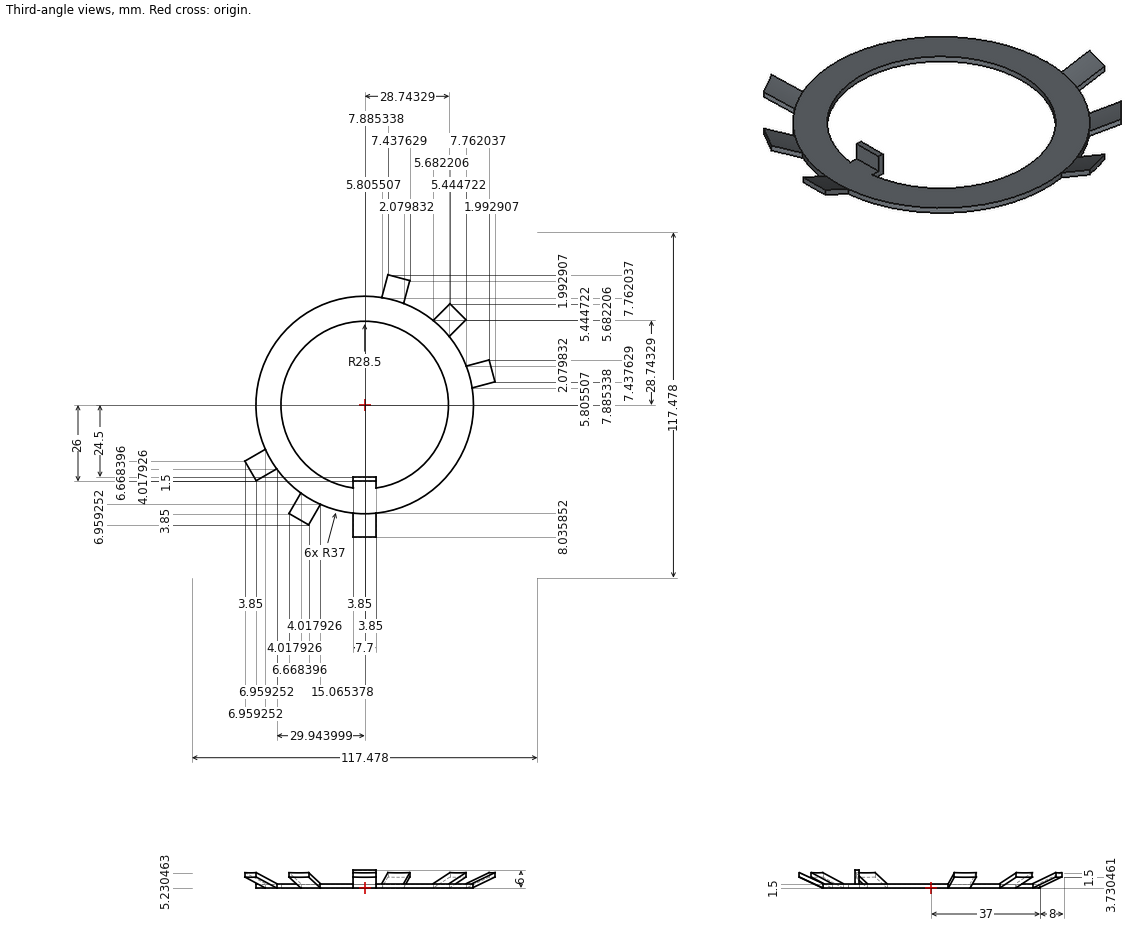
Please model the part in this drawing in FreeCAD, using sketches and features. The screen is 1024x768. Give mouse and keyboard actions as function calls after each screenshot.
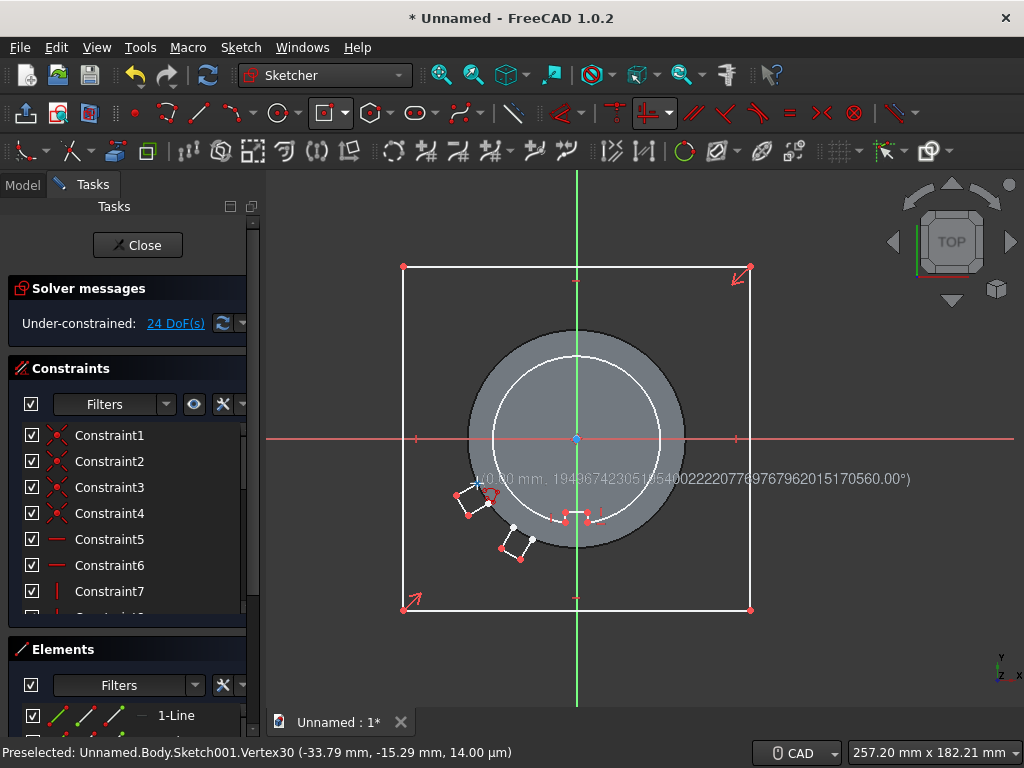
click(594, 331)
click(600, 308)
click(622, 314)
click(616, 337)
right_click(616, 337)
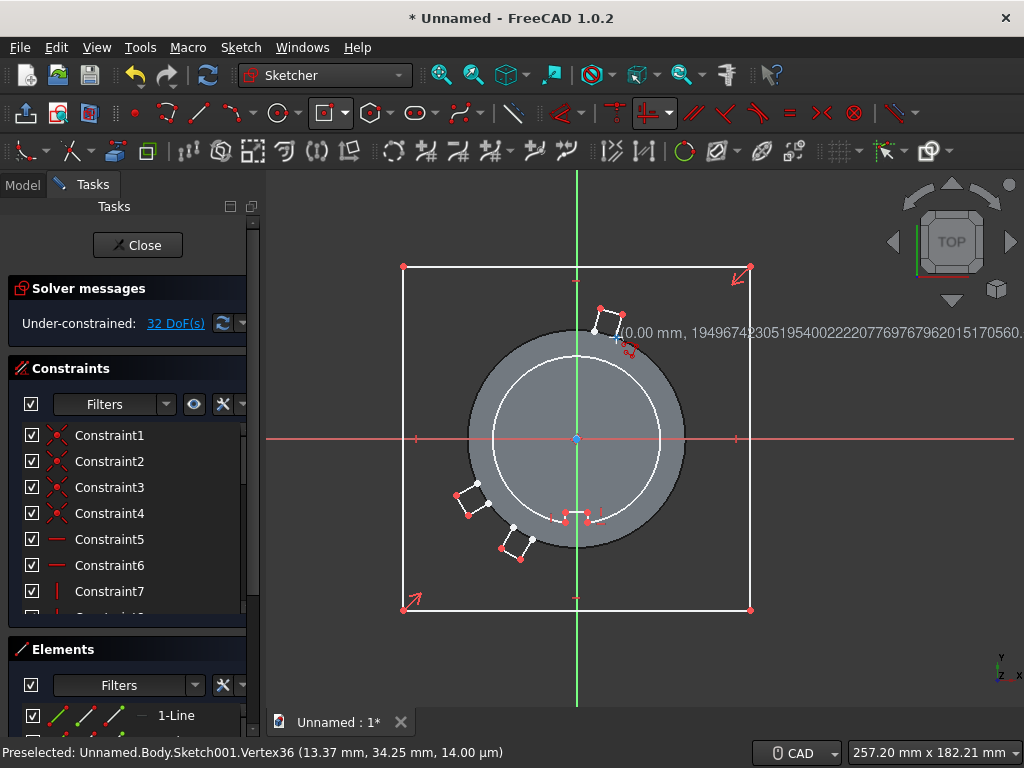
click(645, 354)
click(662, 337)
click(678, 354)
click(661, 370)
right_click(661, 370)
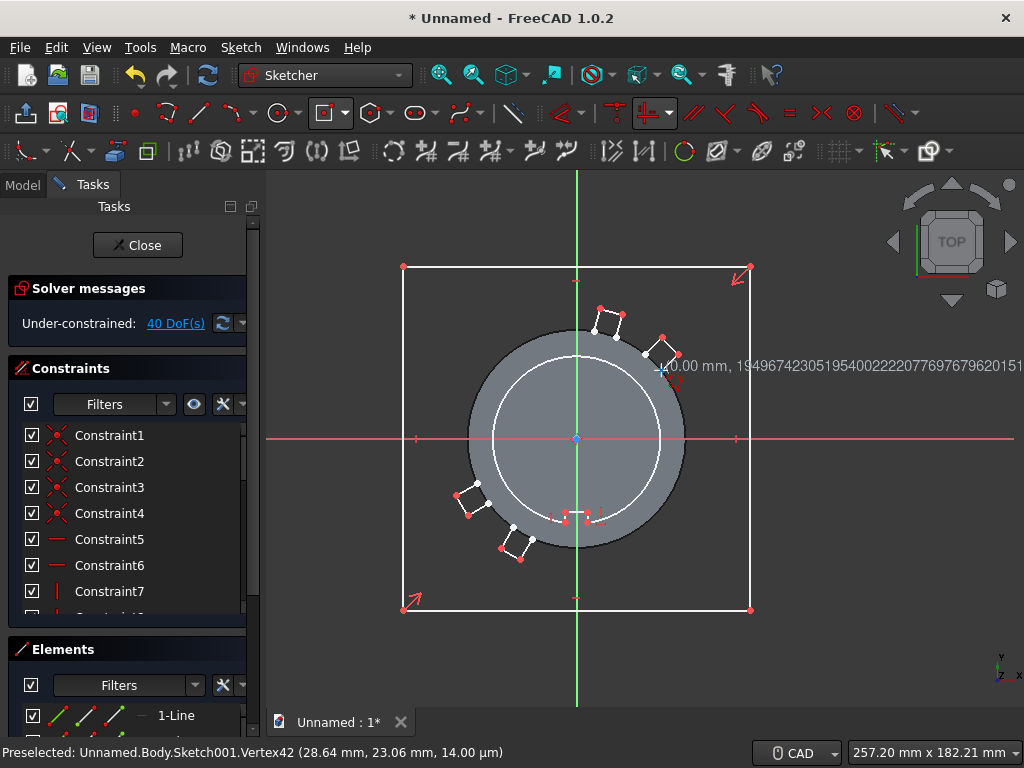
click(678, 400)
click(701, 394)
click(707, 416)
click(684, 422)
right_click(684, 422)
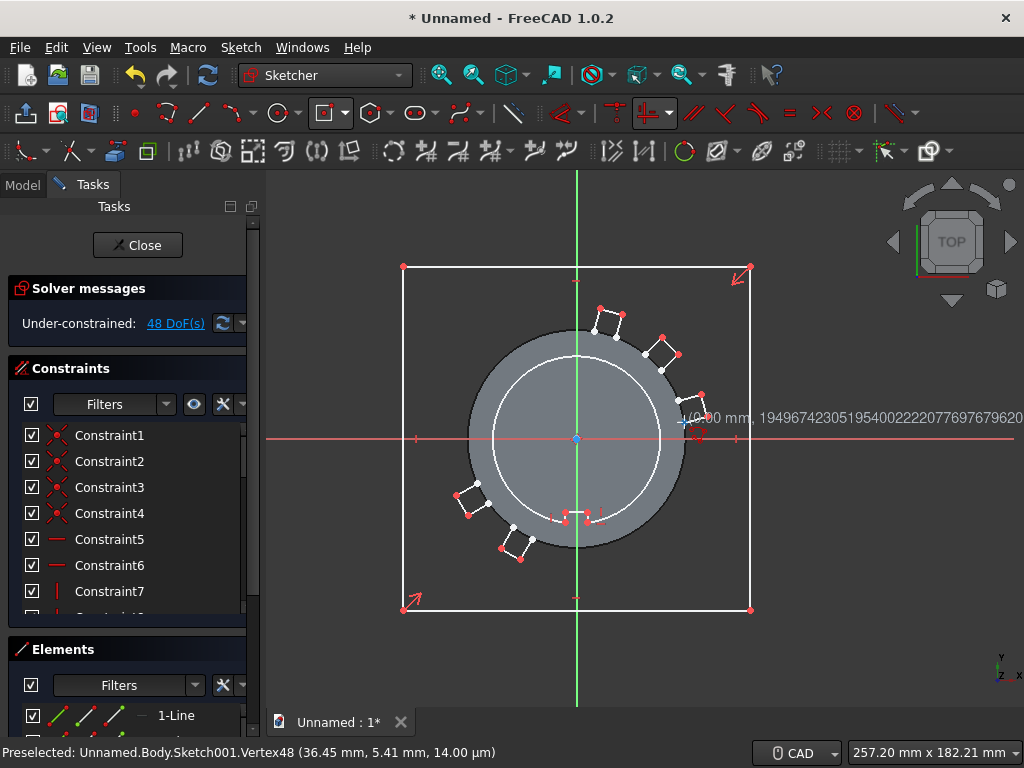
scroll(588, 547, up, 2)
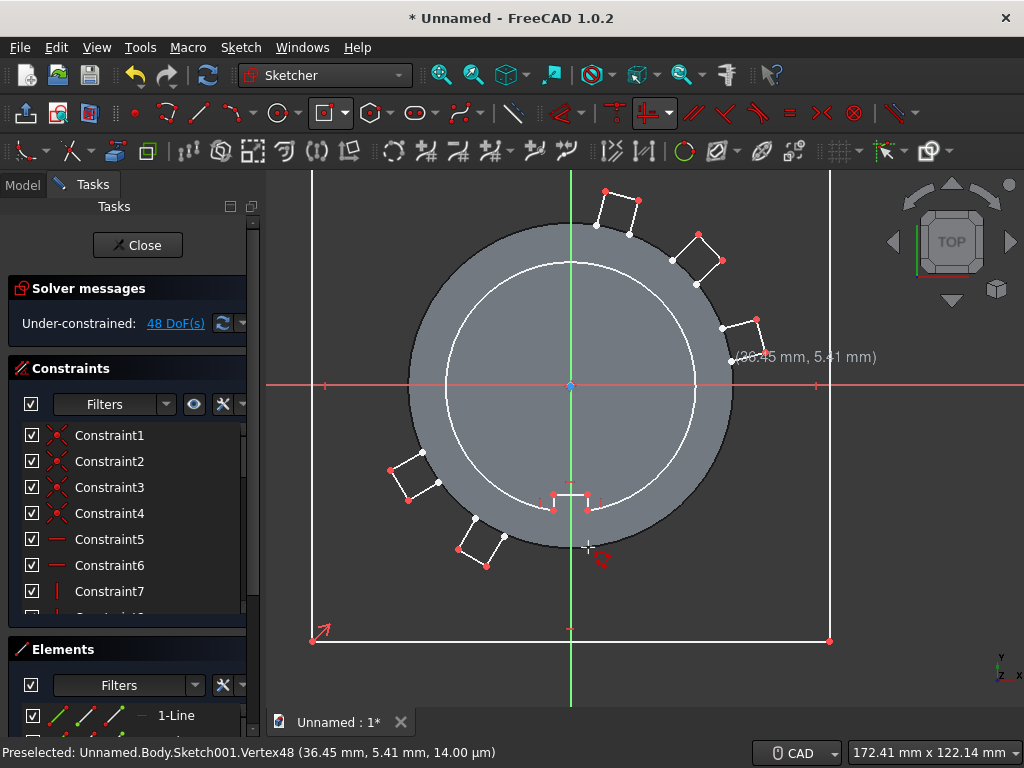
click(588, 547)
click(588, 583)
click(554, 583)
click(554, 547)
right_click(554, 547)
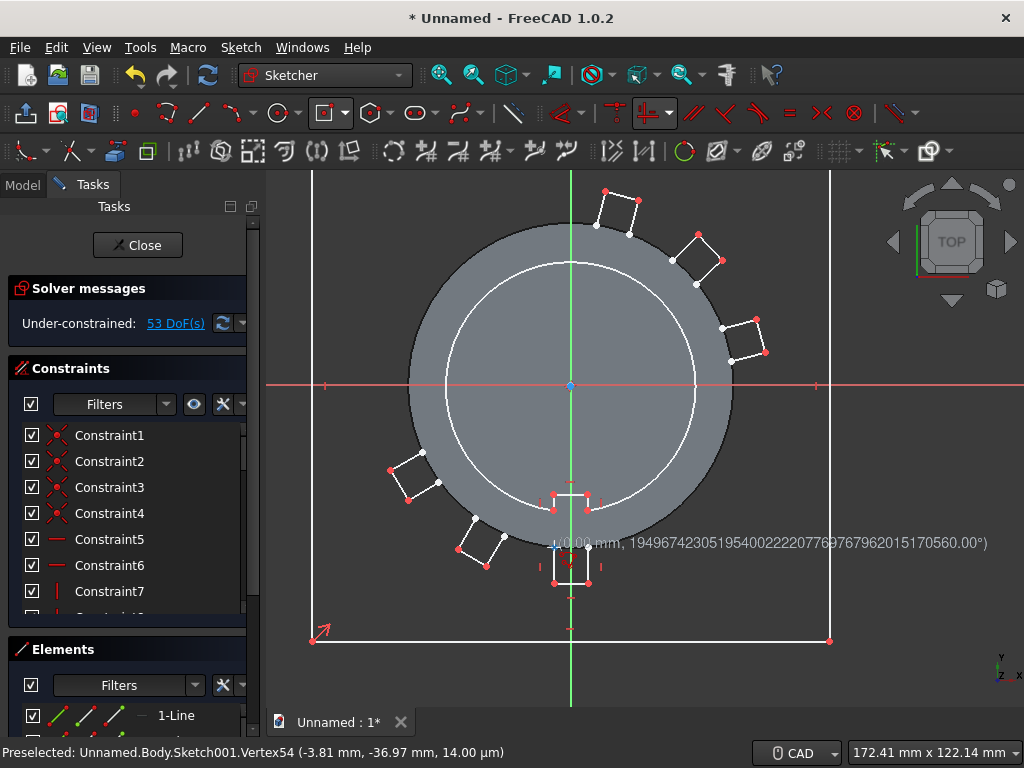
click(232, 114)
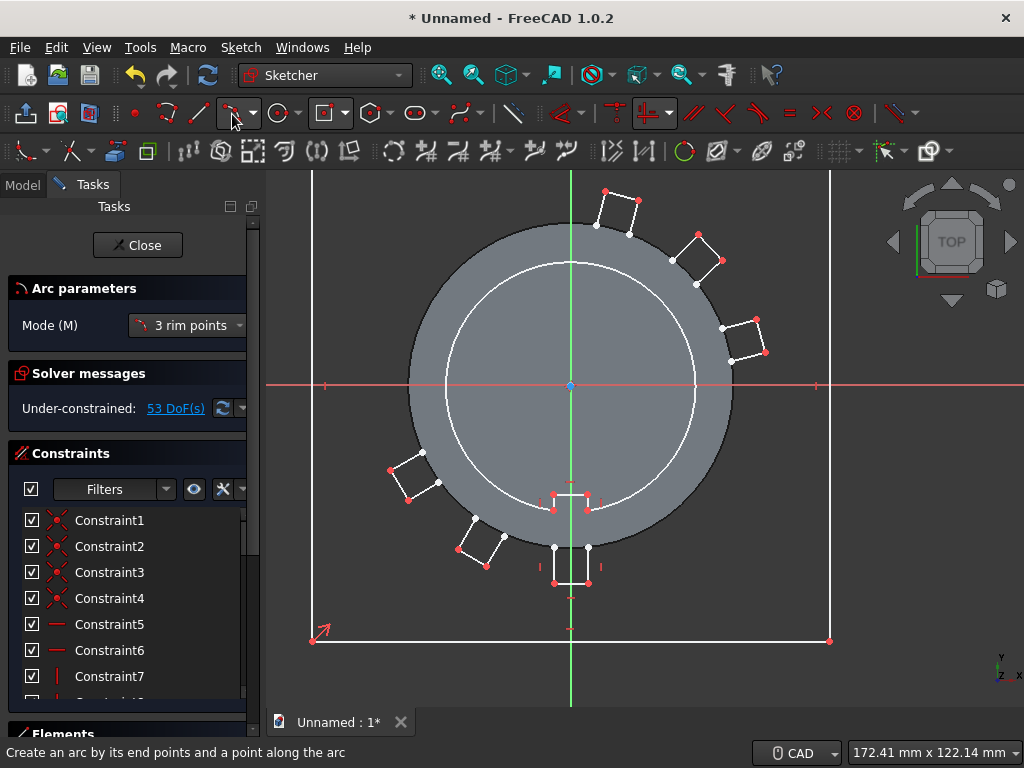
click(476, 518)
click(439, 483)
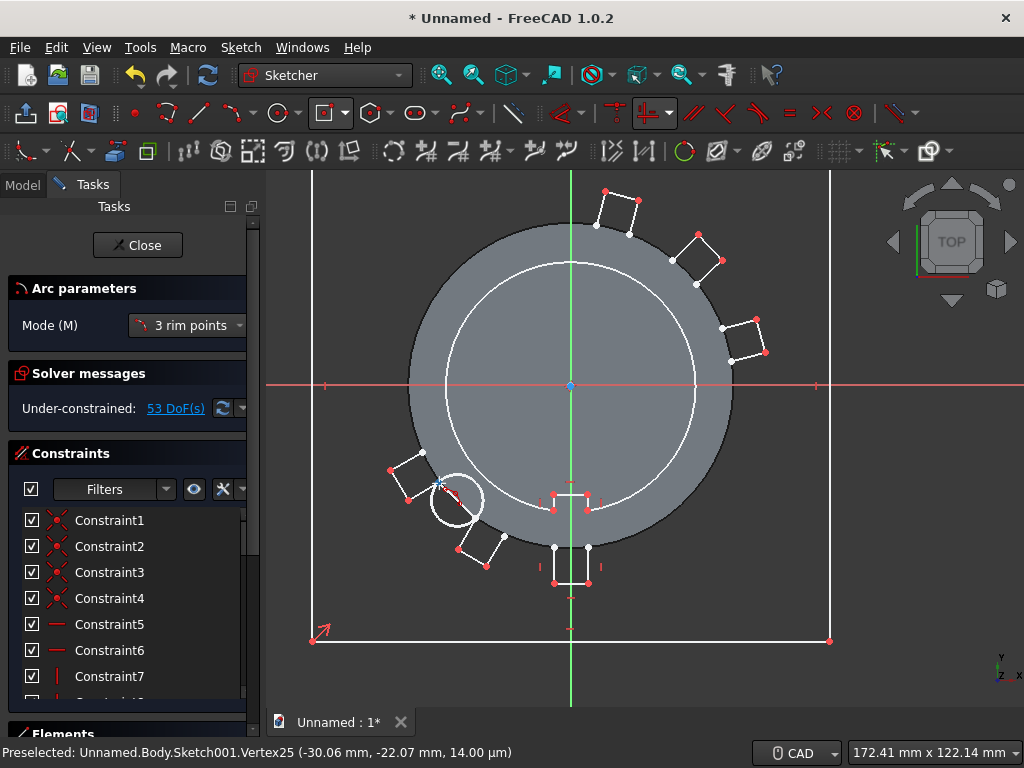
scroll(456, 500, up, 11)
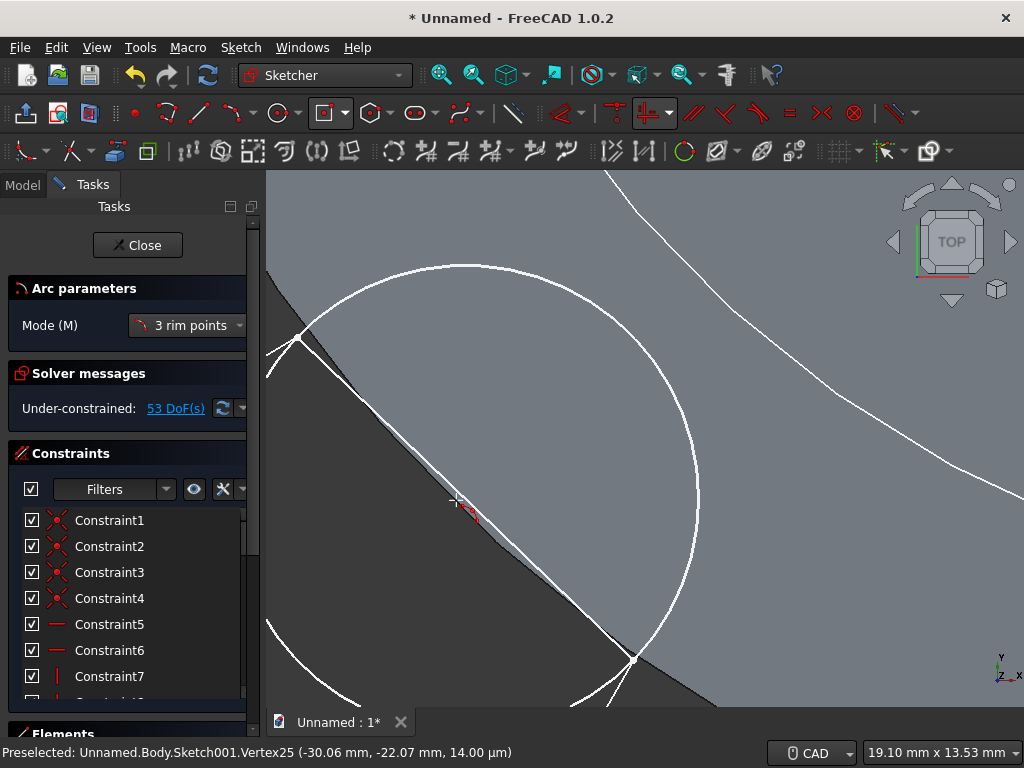
click(452, 500)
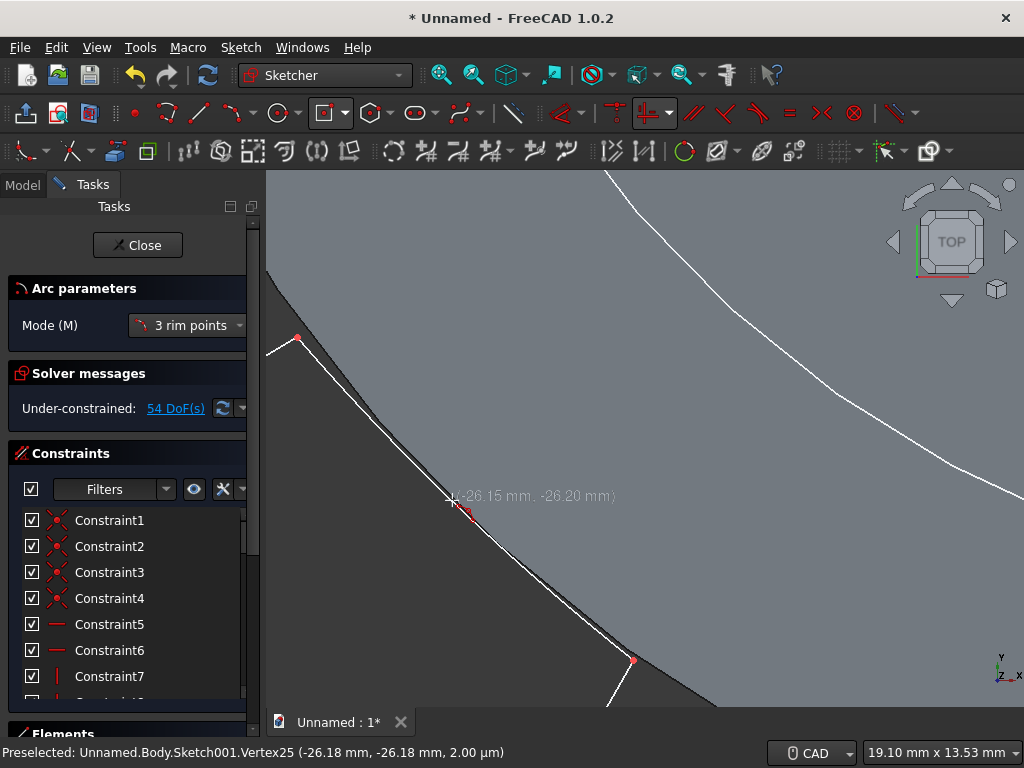
scroll(503, 517, down, 13)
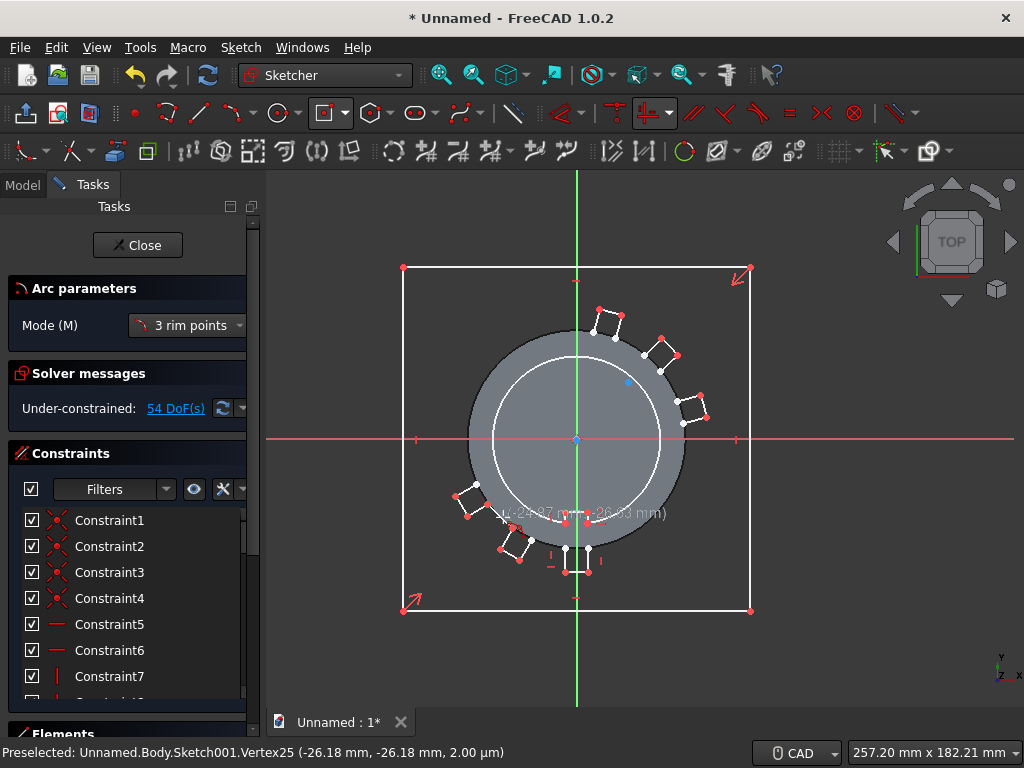
scroll(477, 484, up, 2)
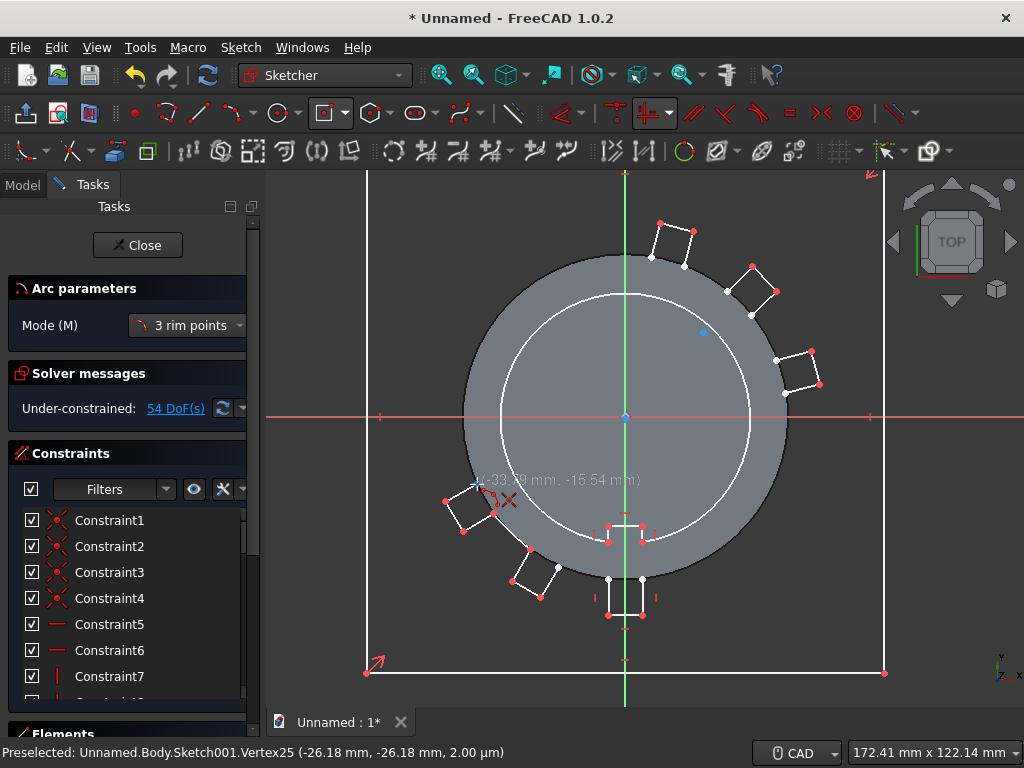
click(477, 484)
click(651, 257)
click(496, 318)